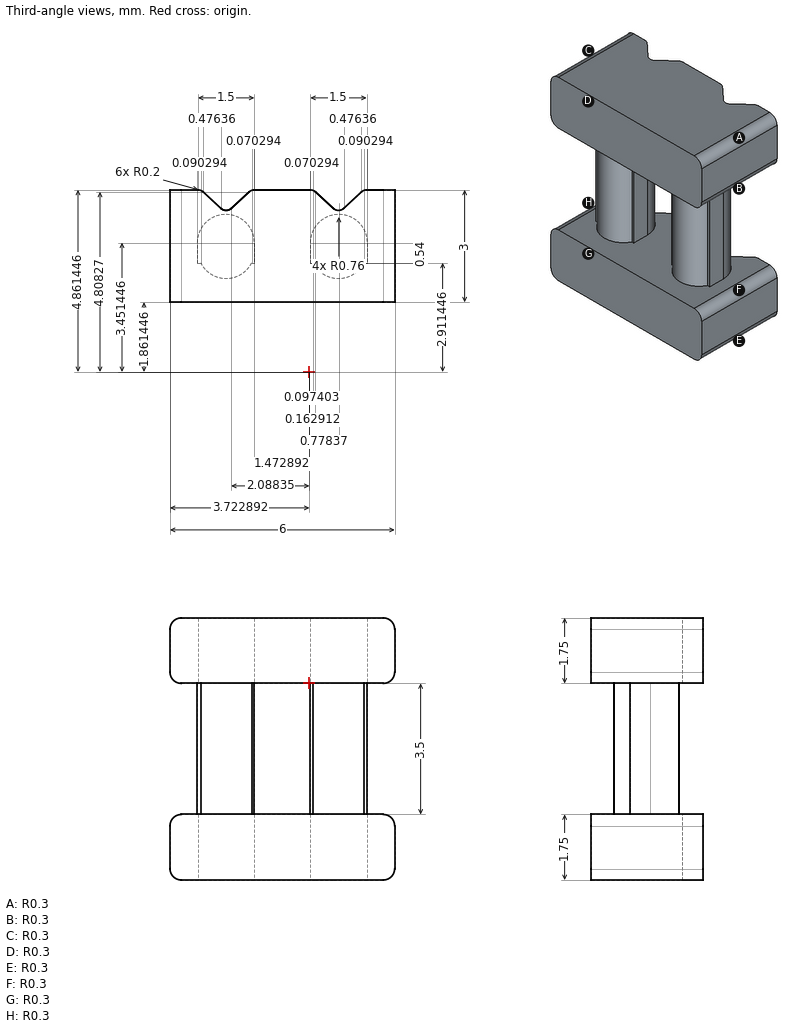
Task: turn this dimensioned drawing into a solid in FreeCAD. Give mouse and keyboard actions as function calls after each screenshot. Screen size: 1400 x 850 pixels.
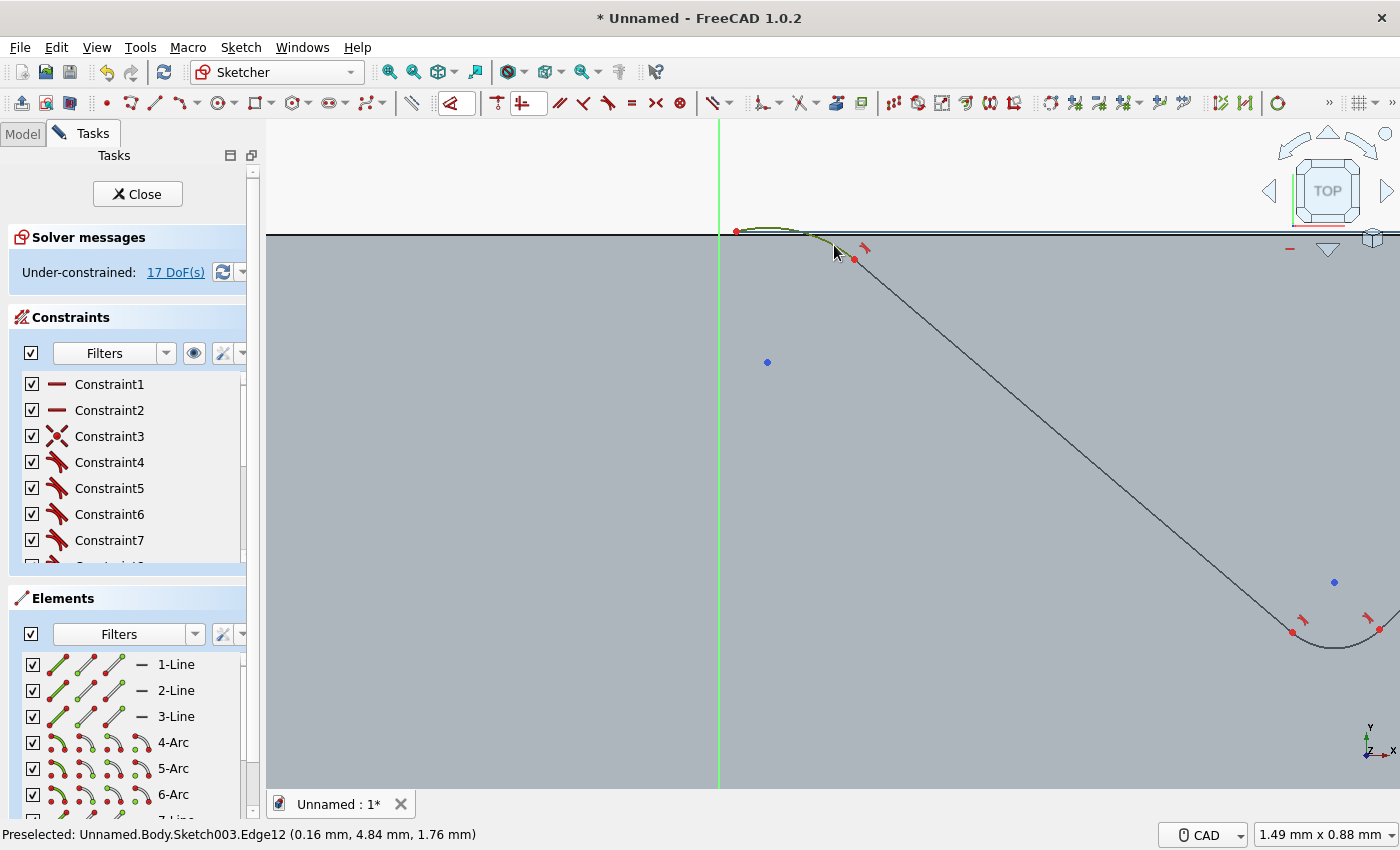
click(608, 104)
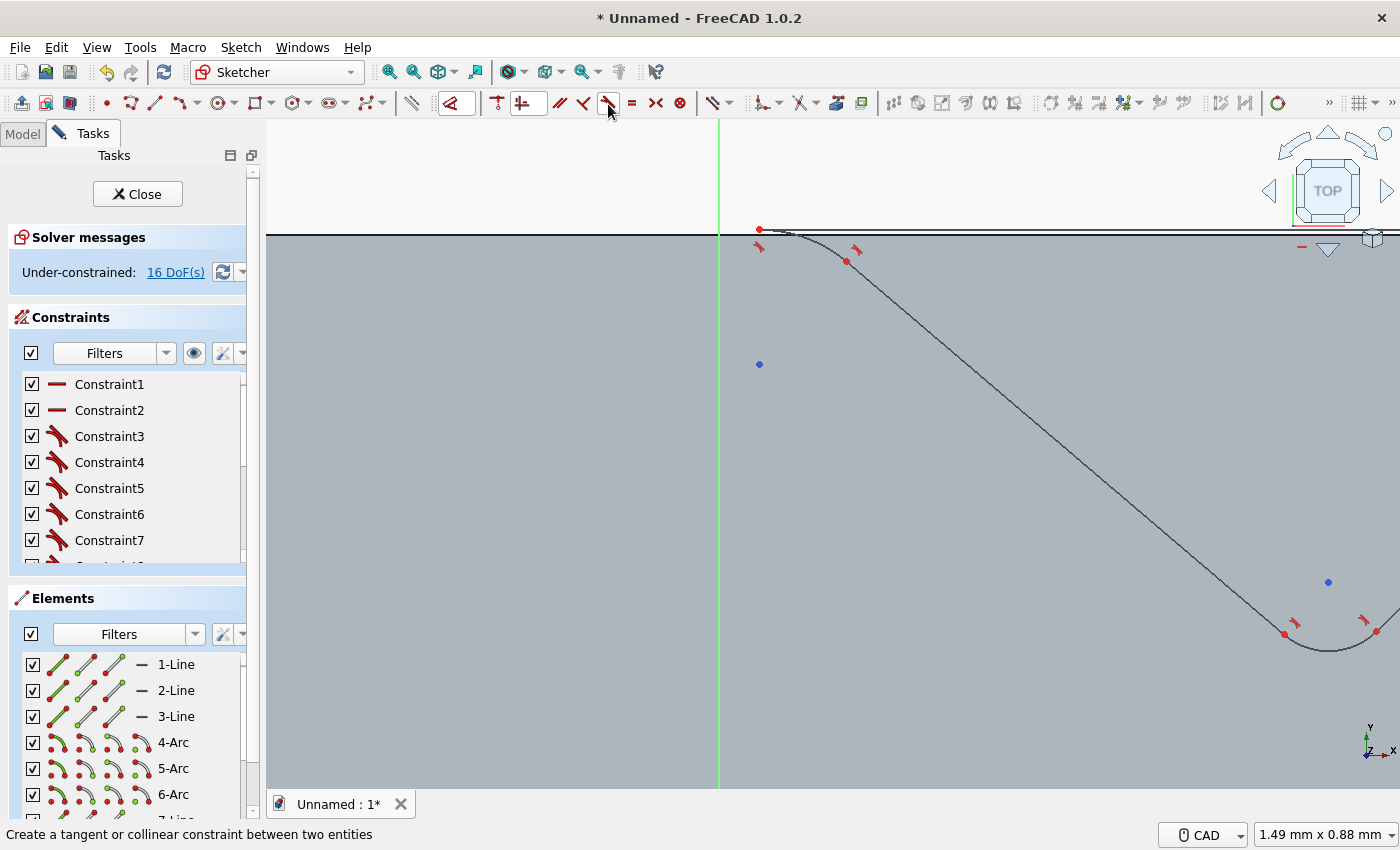
scroll(839, 251, down, 11)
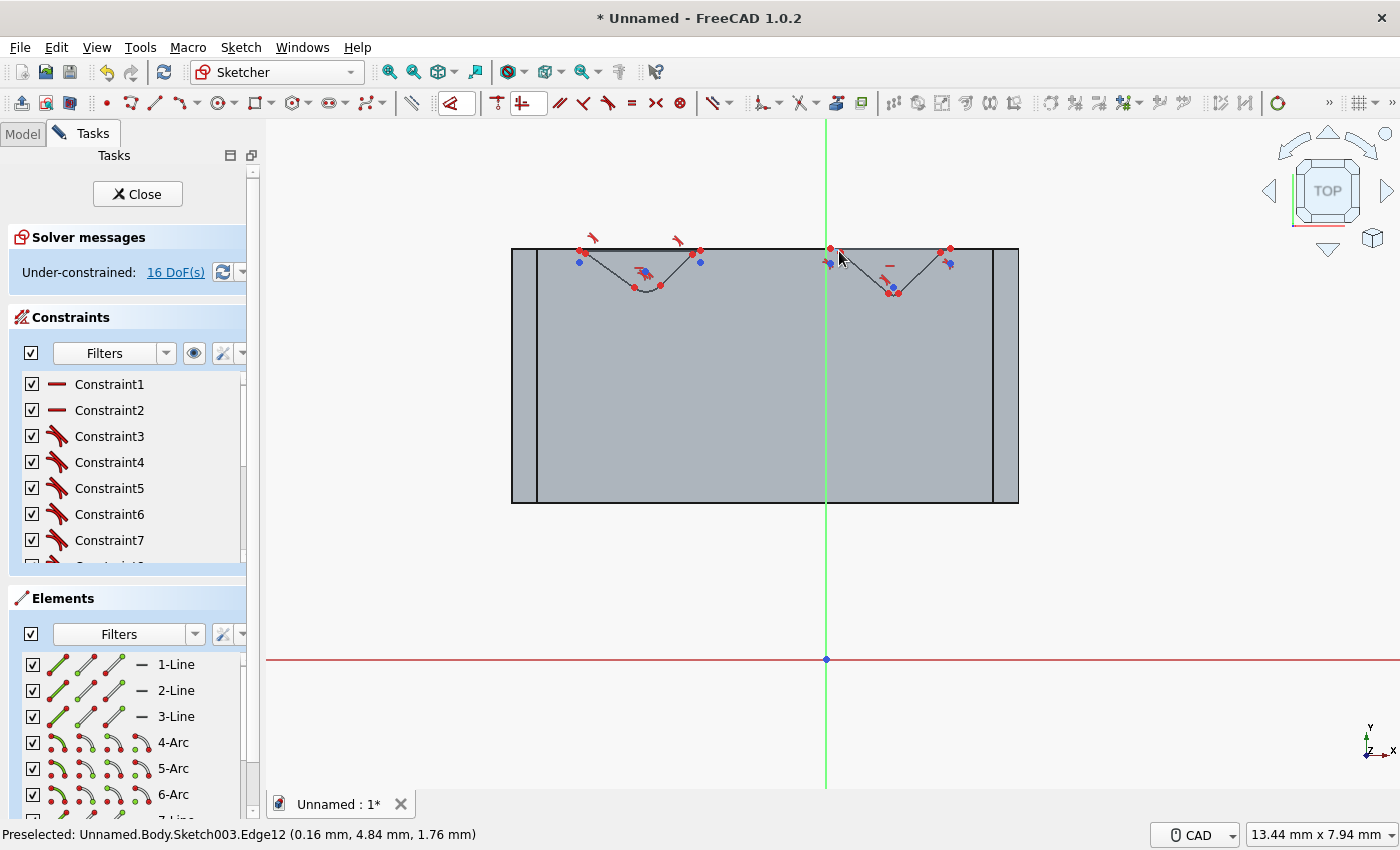
scroll(584, 252, up, 13)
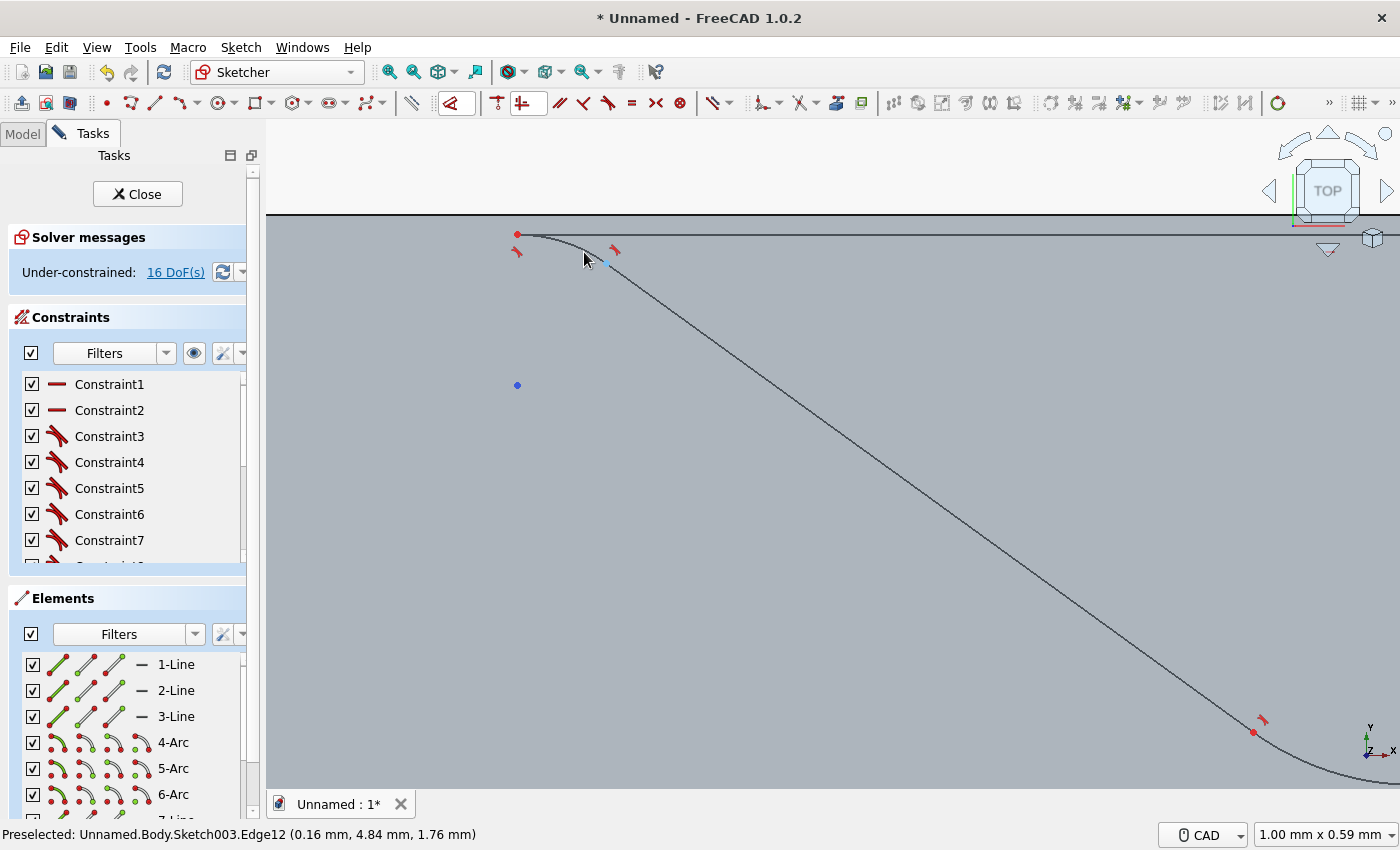
click(582, 249)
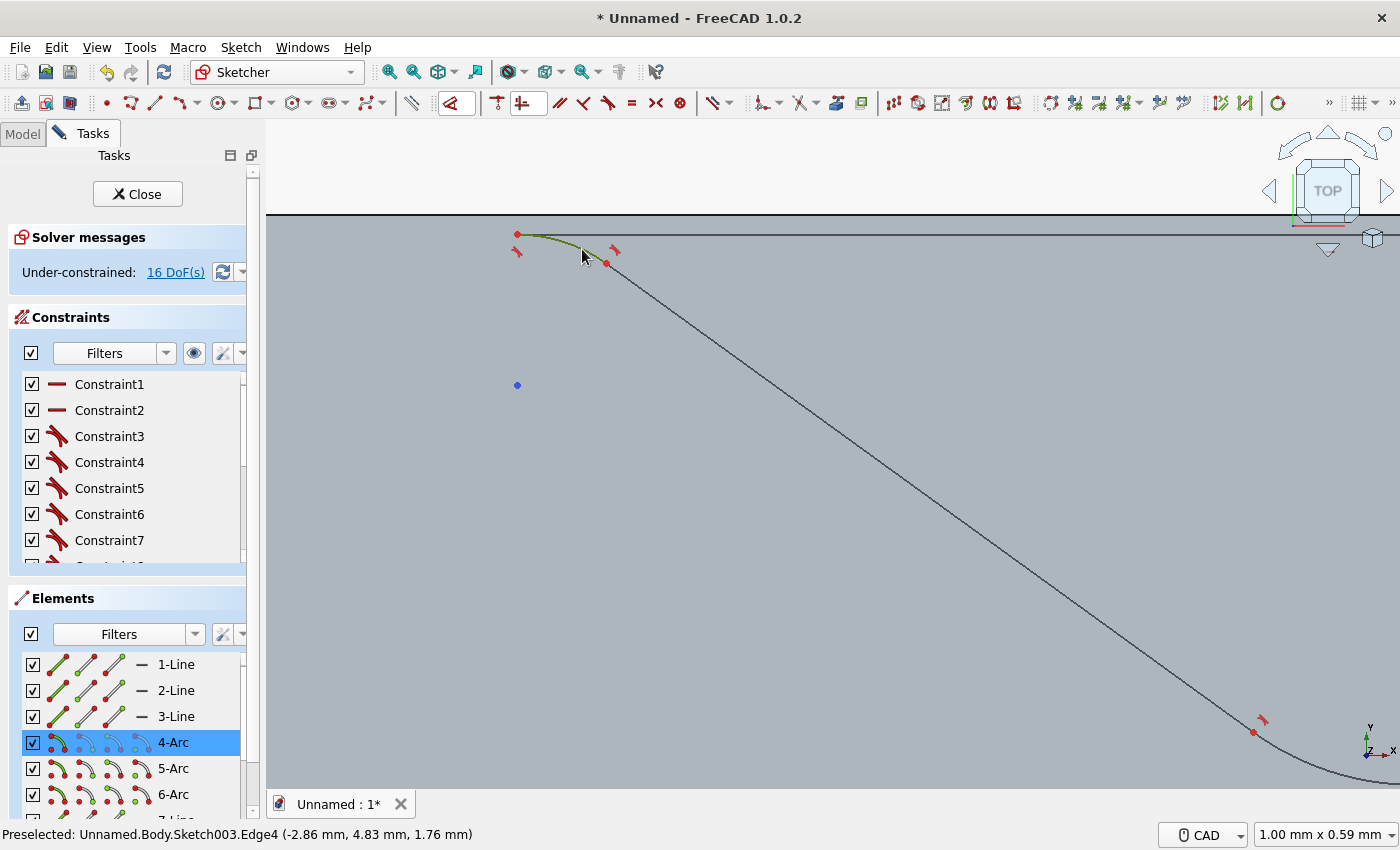
scroll(584, 252, down, 13)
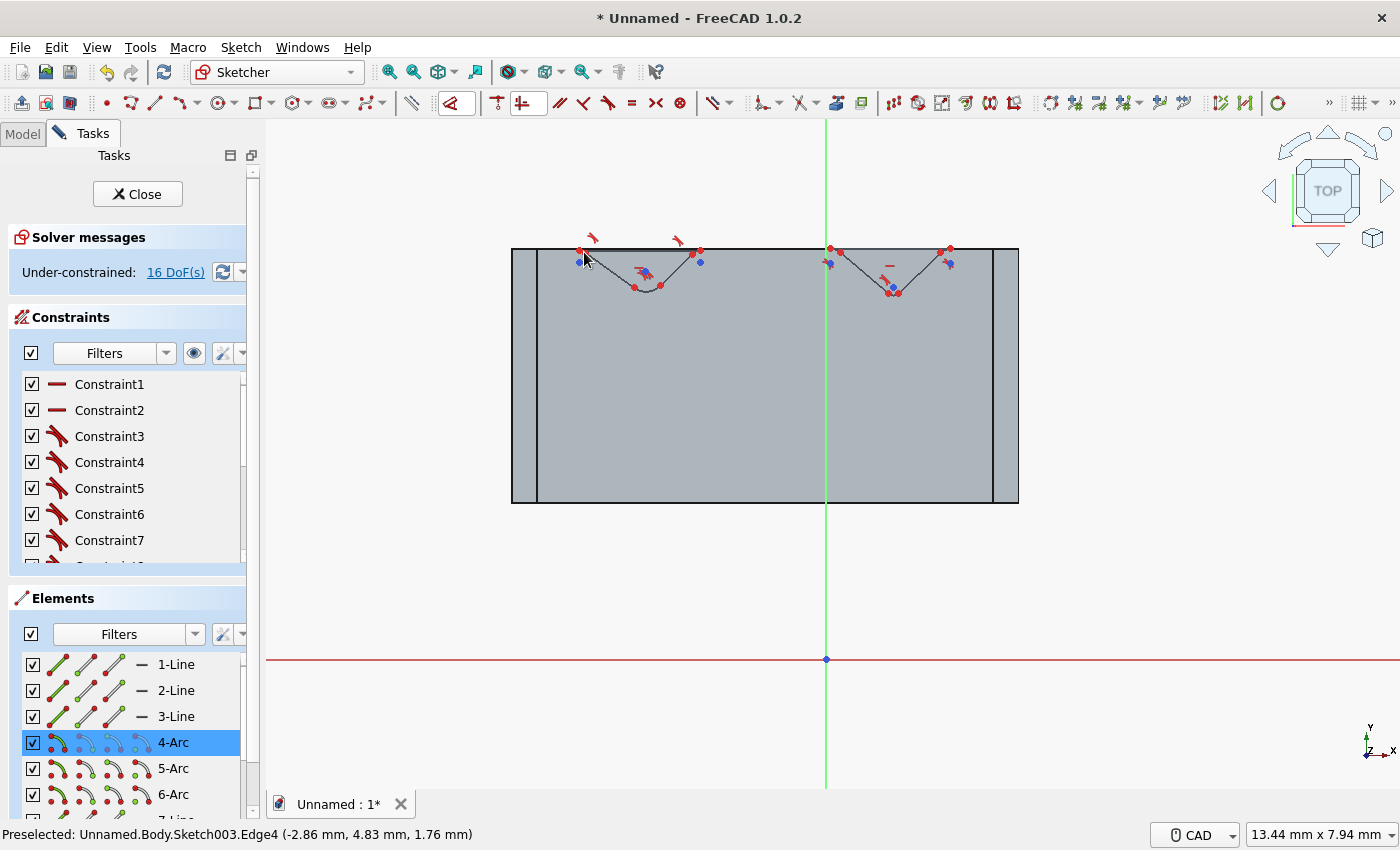
scroll(642, 291, up, 3)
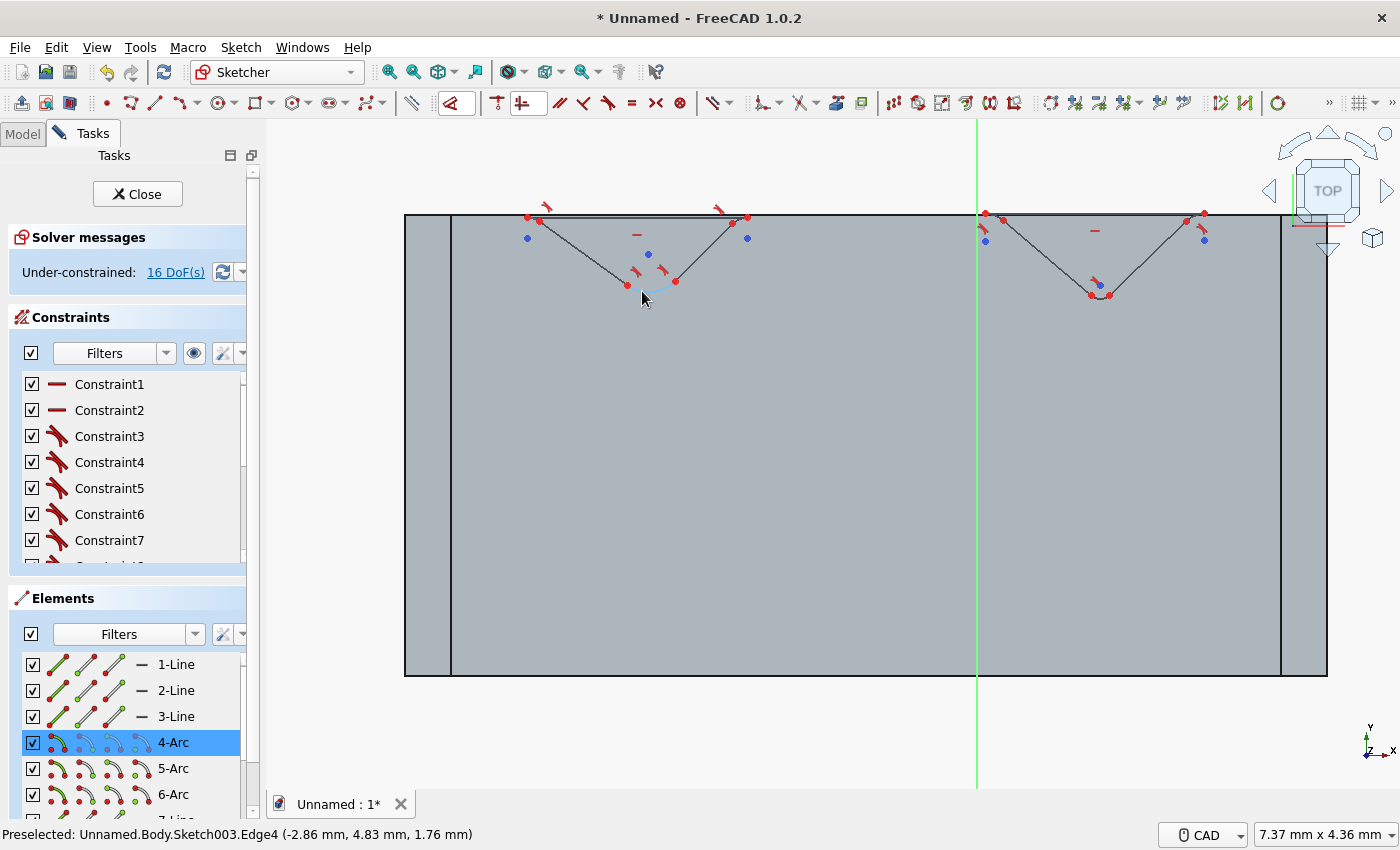
click(641, 291)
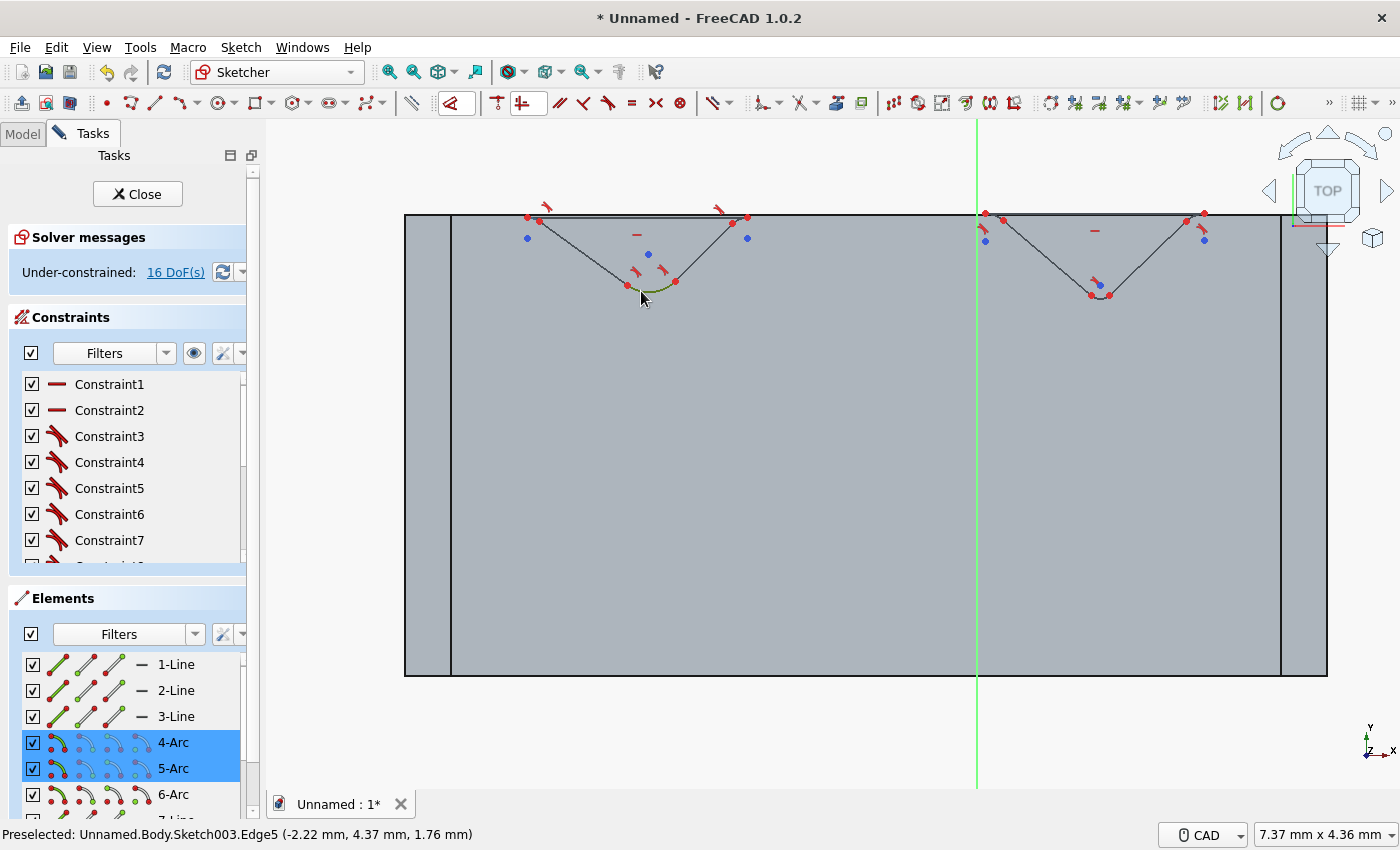
scroll(735, 222, up, 8)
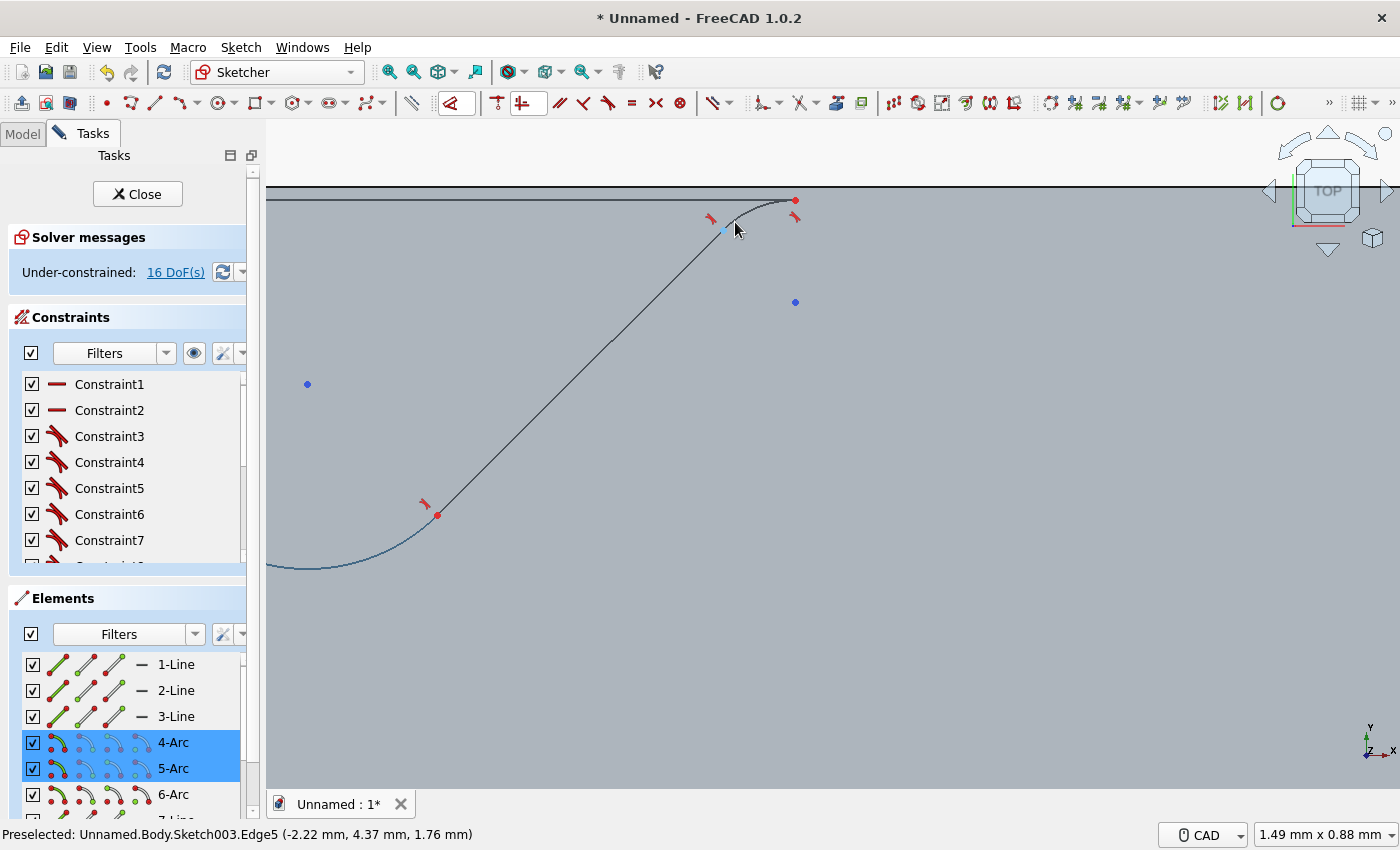
click(735, 220)